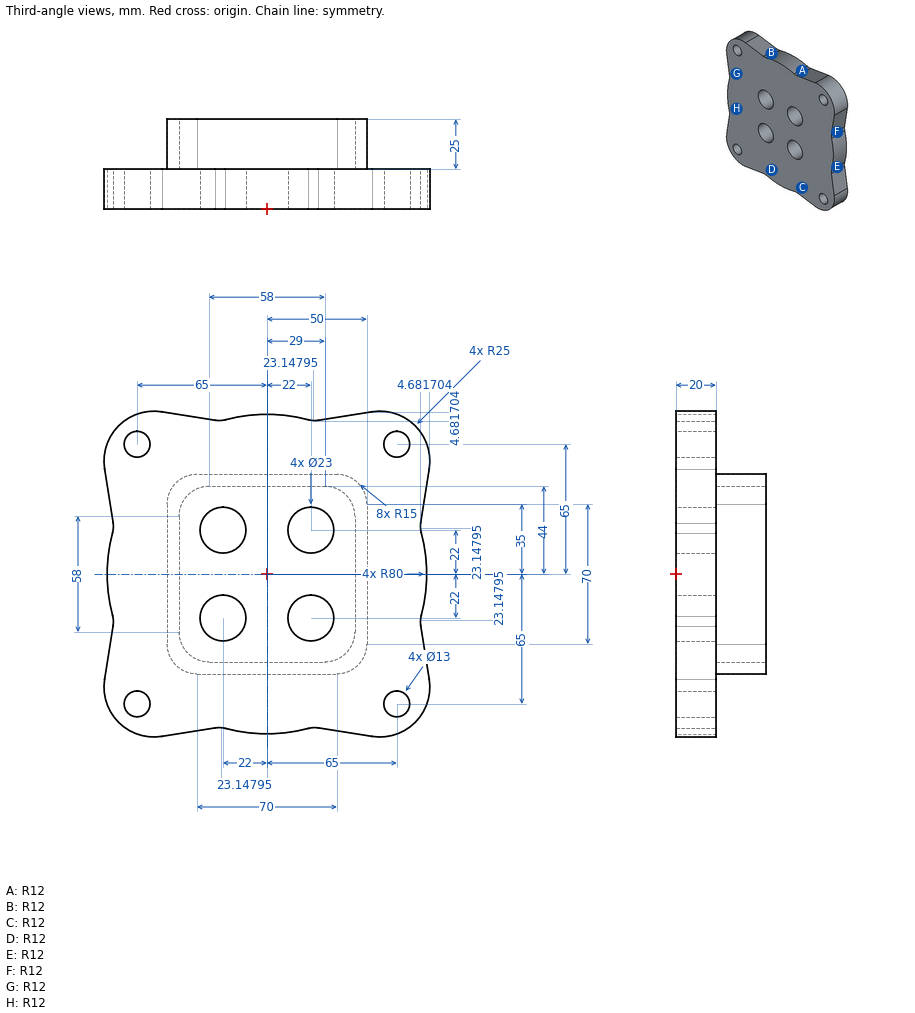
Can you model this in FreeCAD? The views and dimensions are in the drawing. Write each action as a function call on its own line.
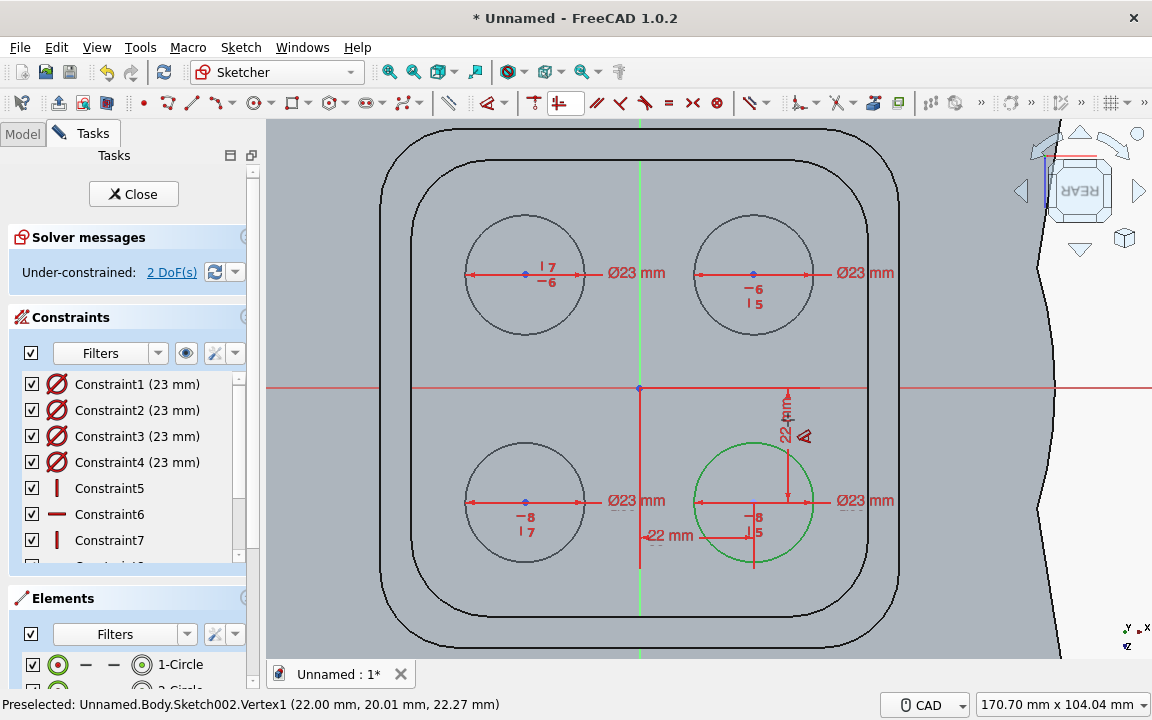
click(754, 275)
click(788, 306)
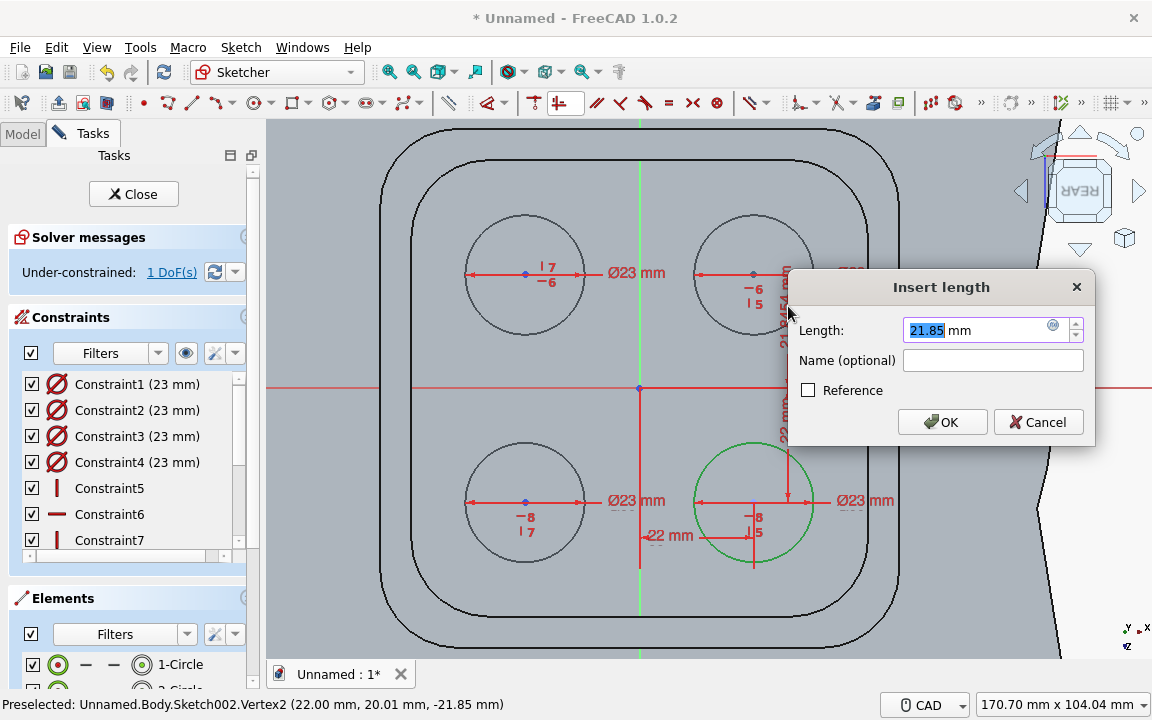
text(22)
key(Return)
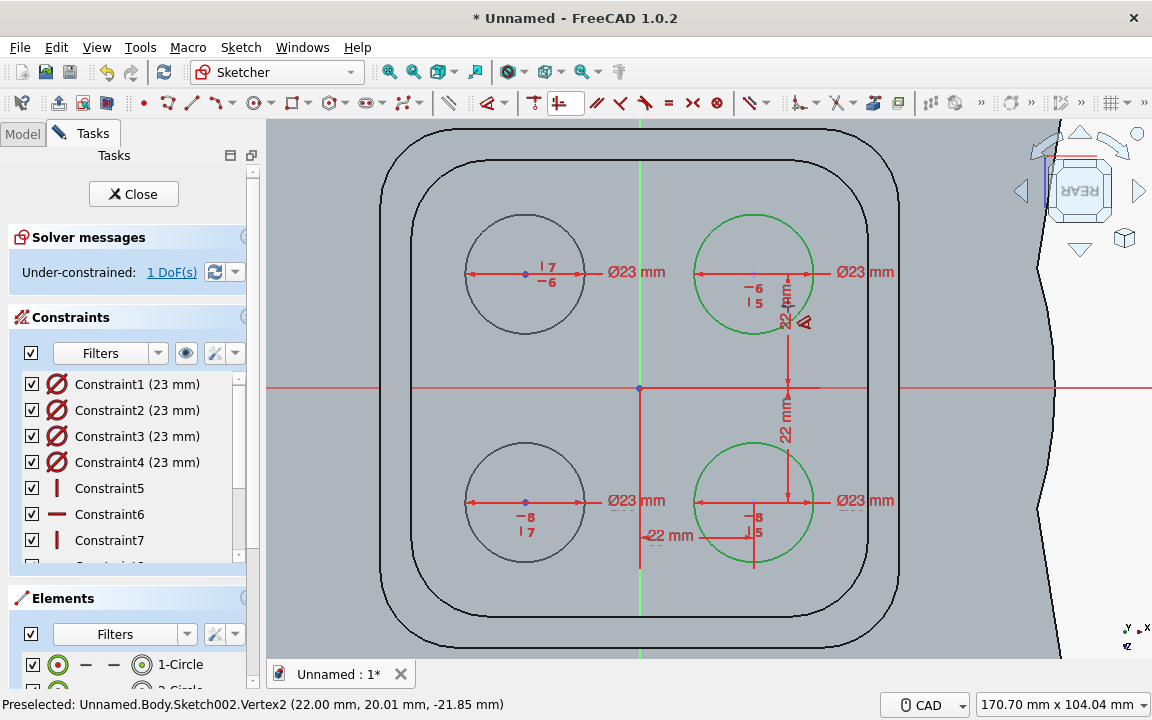
click(525, 274)
click(556, 240)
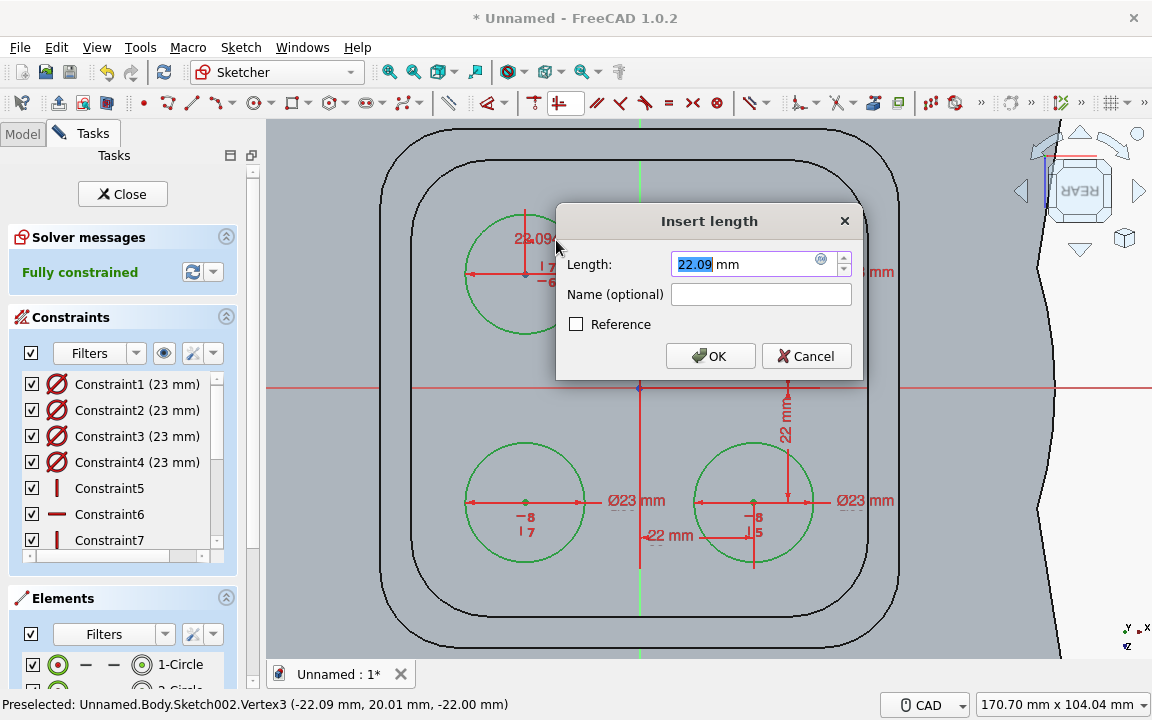
text(22)
key(Return)
key(Escape)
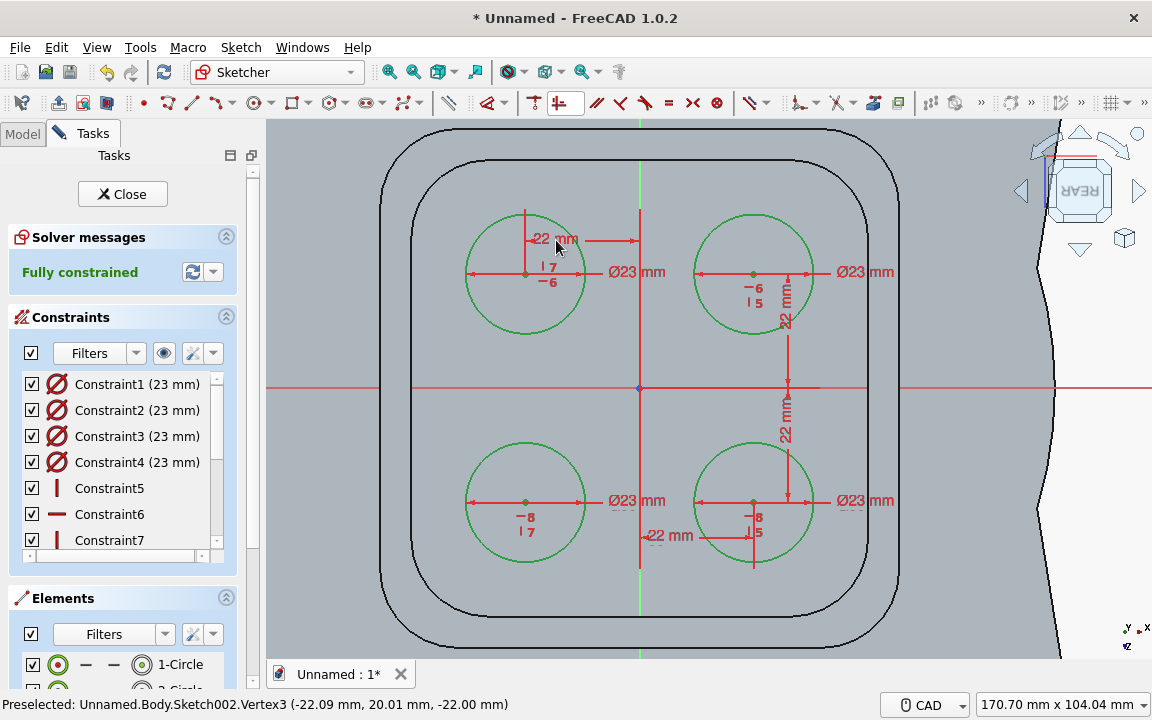
click(123, 194)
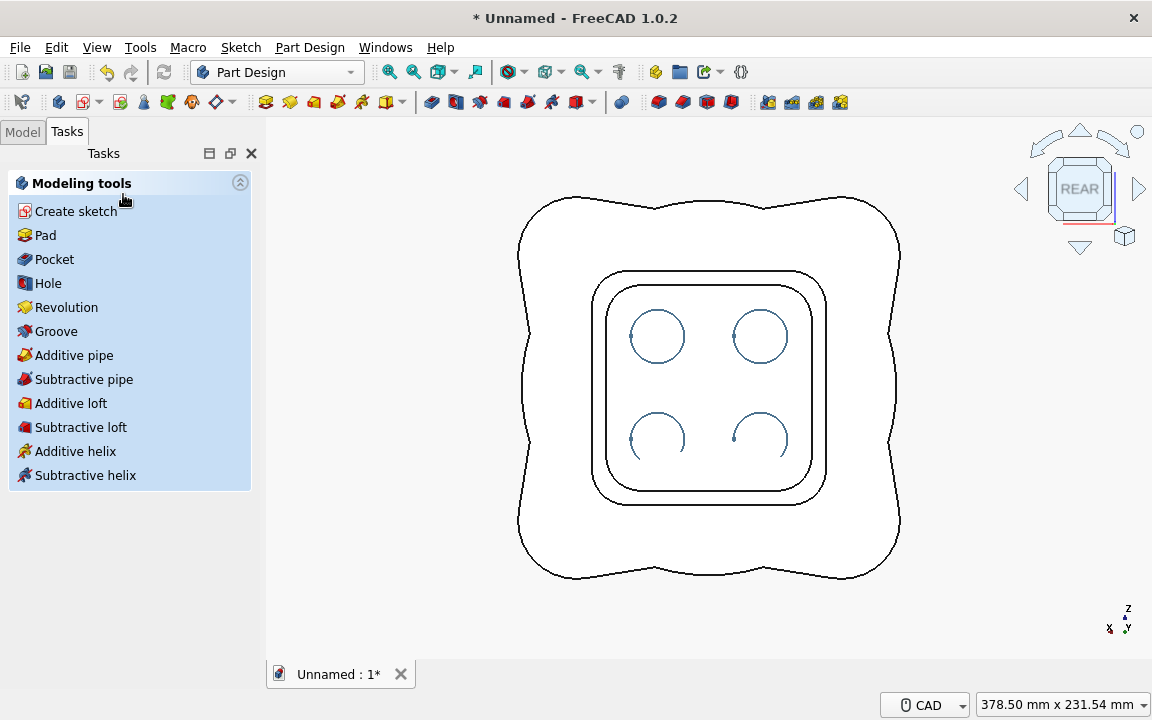
click(432, 102)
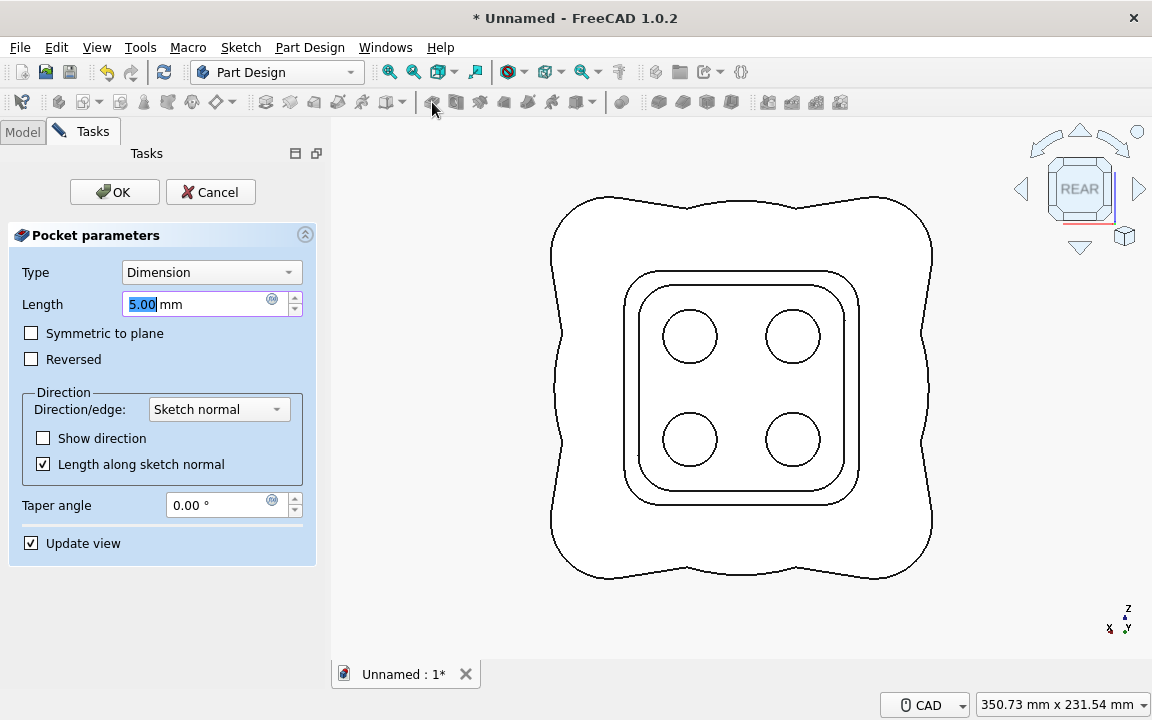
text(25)
key(Tab)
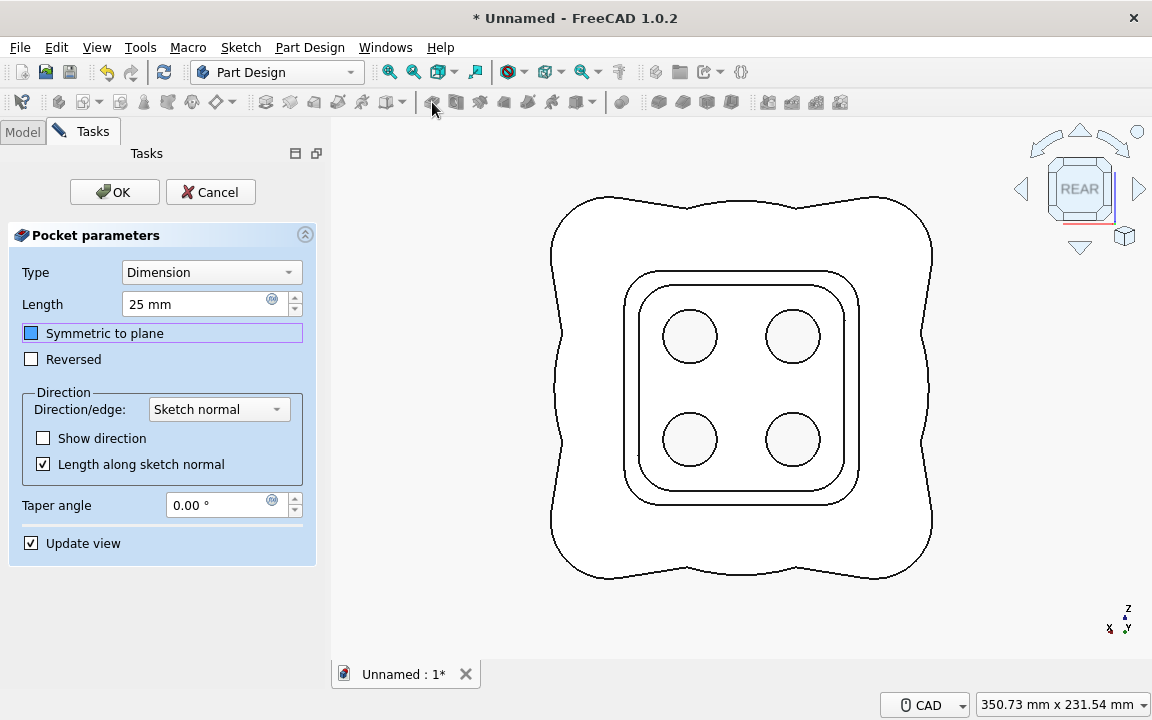
click(115, 192)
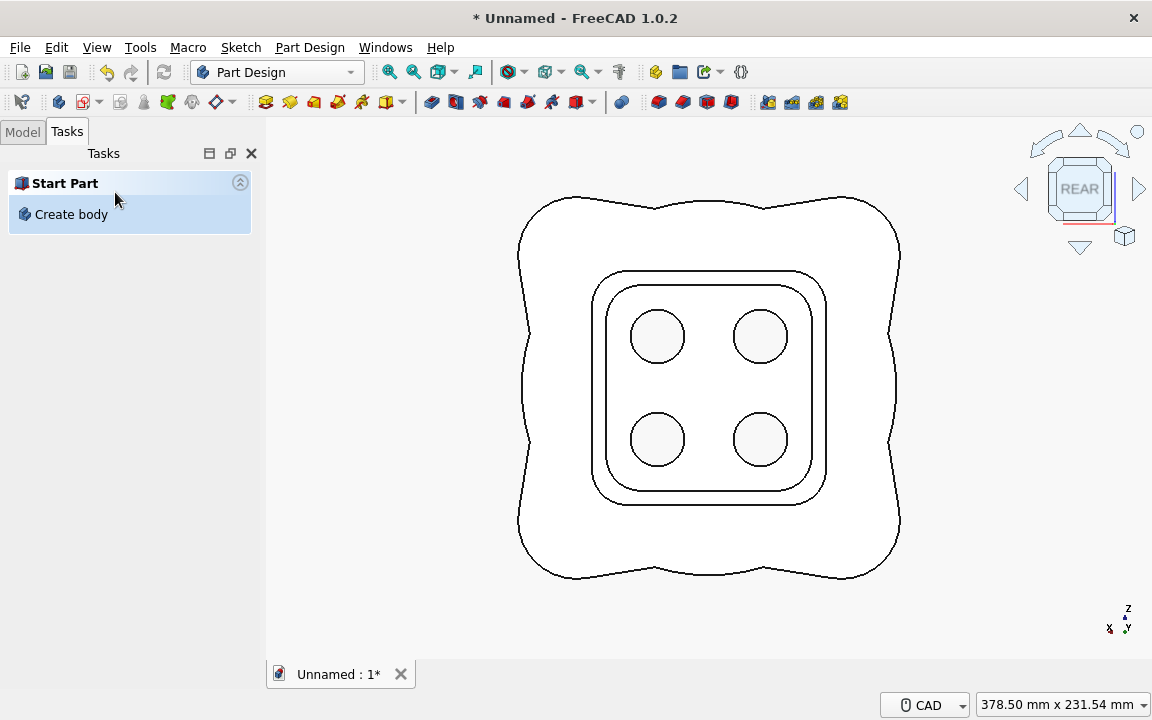
key(0)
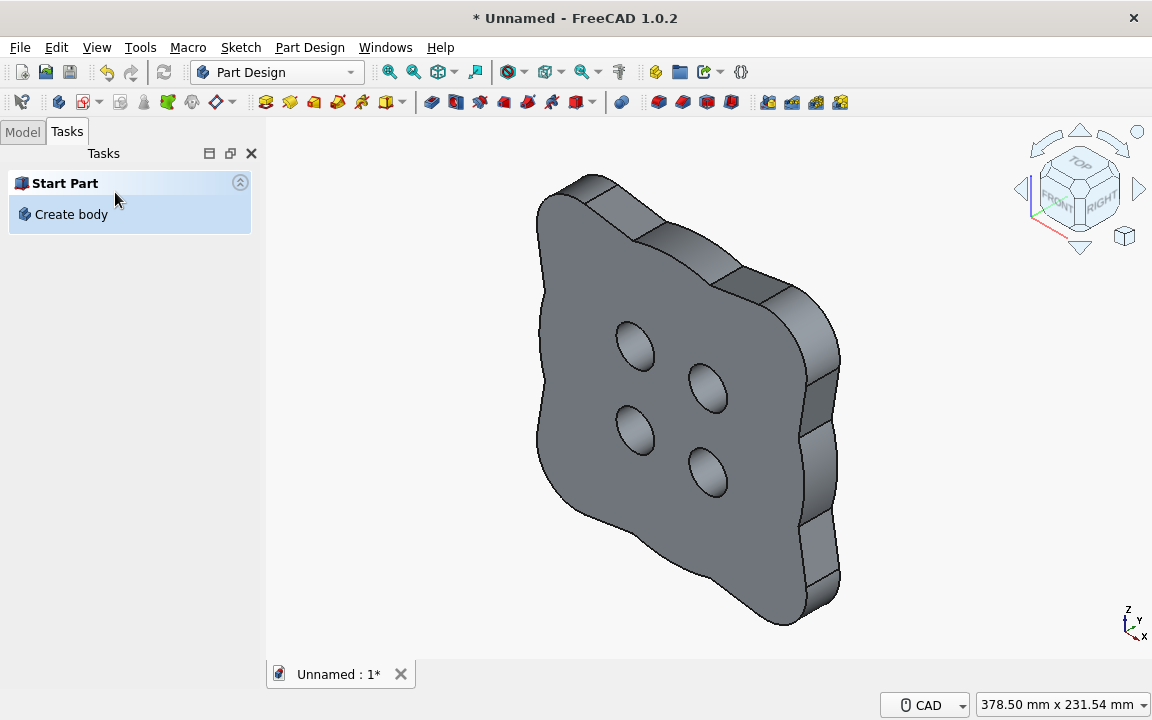
key(2)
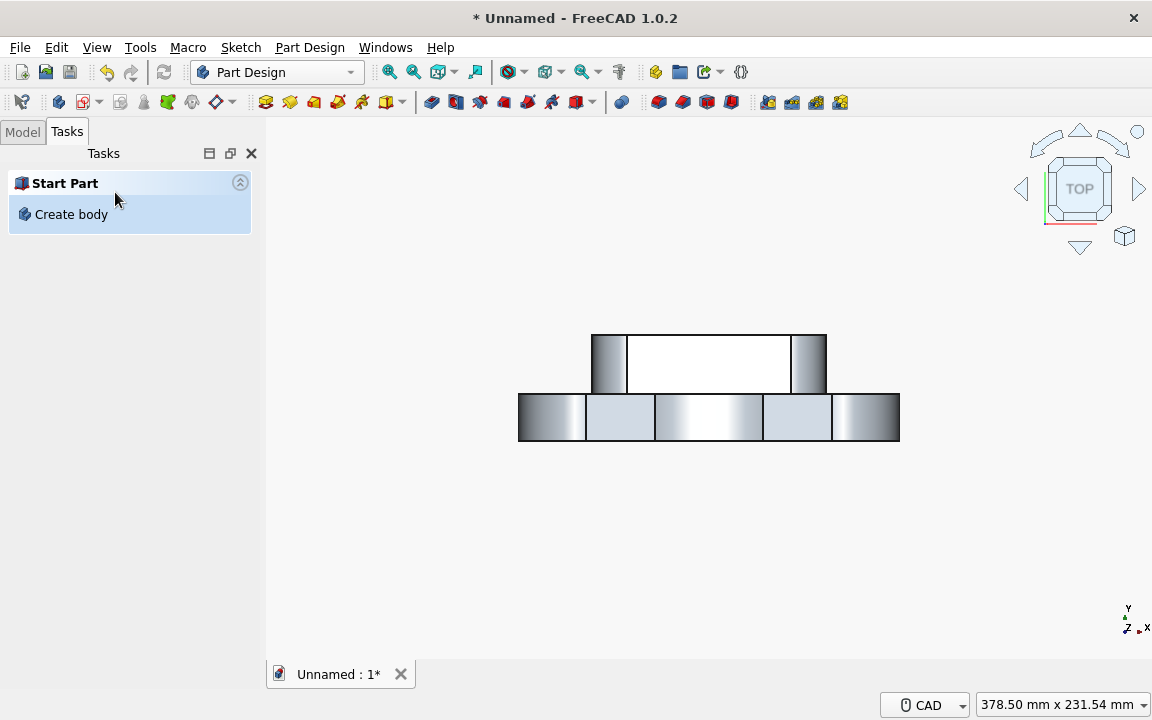
click(390, 72)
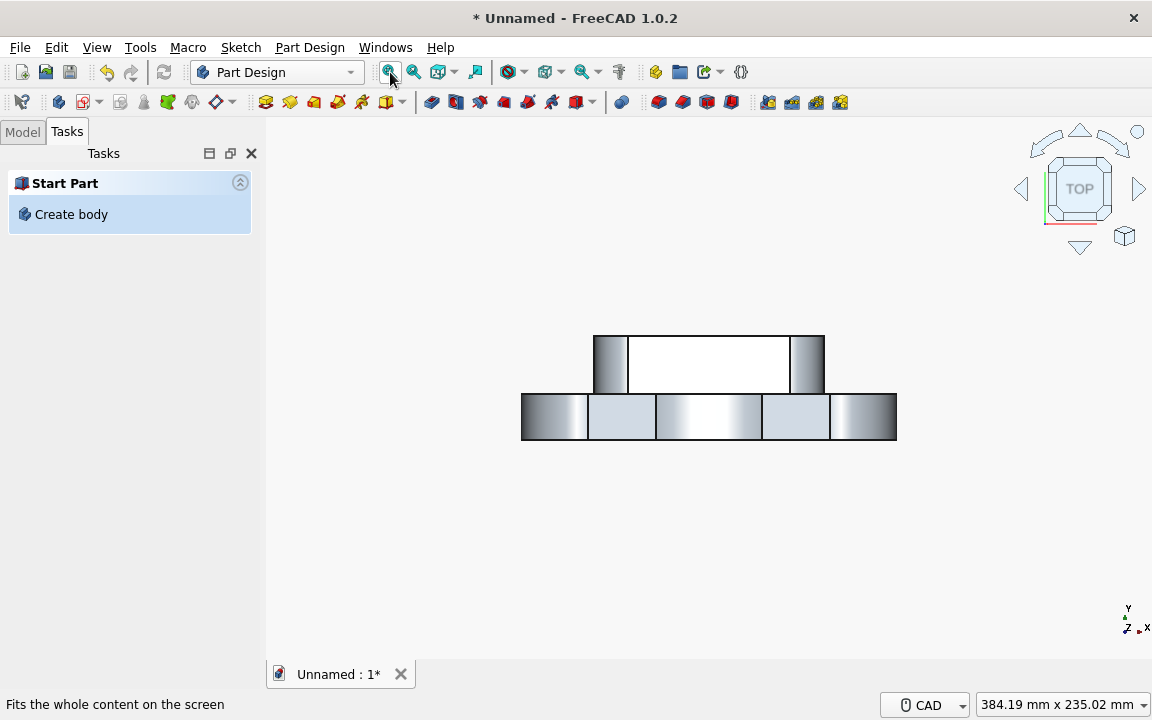
key(1)